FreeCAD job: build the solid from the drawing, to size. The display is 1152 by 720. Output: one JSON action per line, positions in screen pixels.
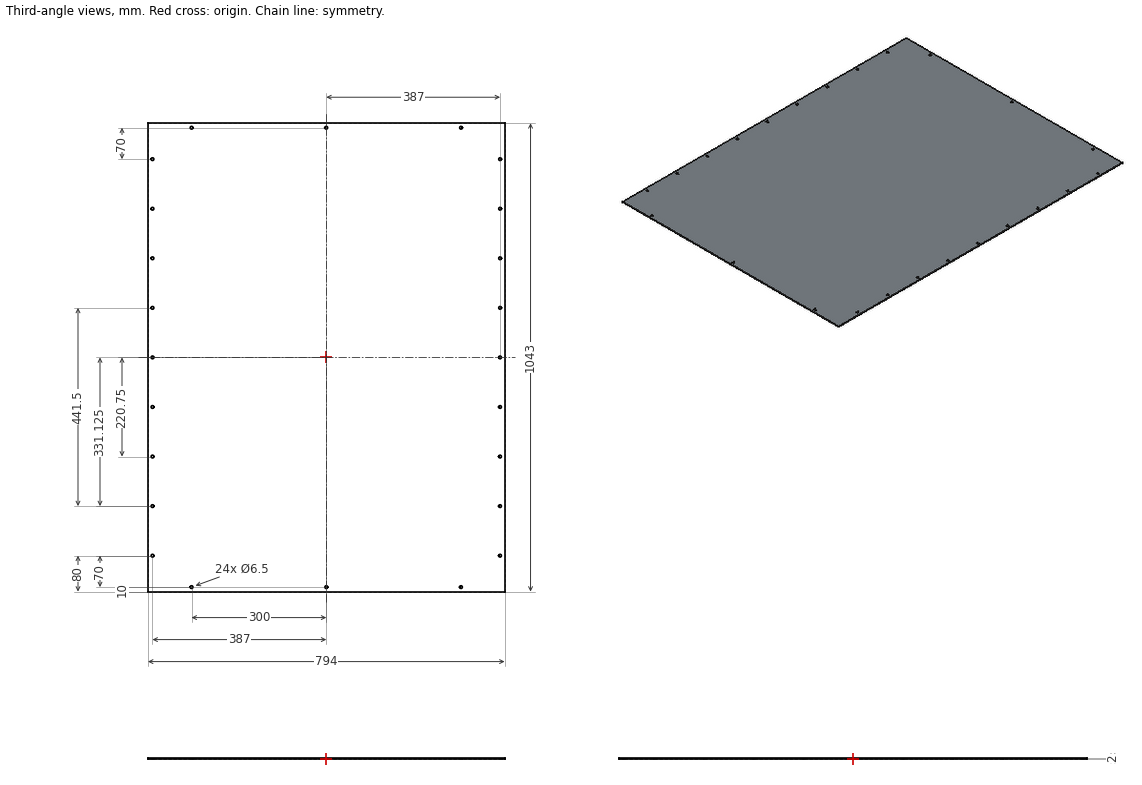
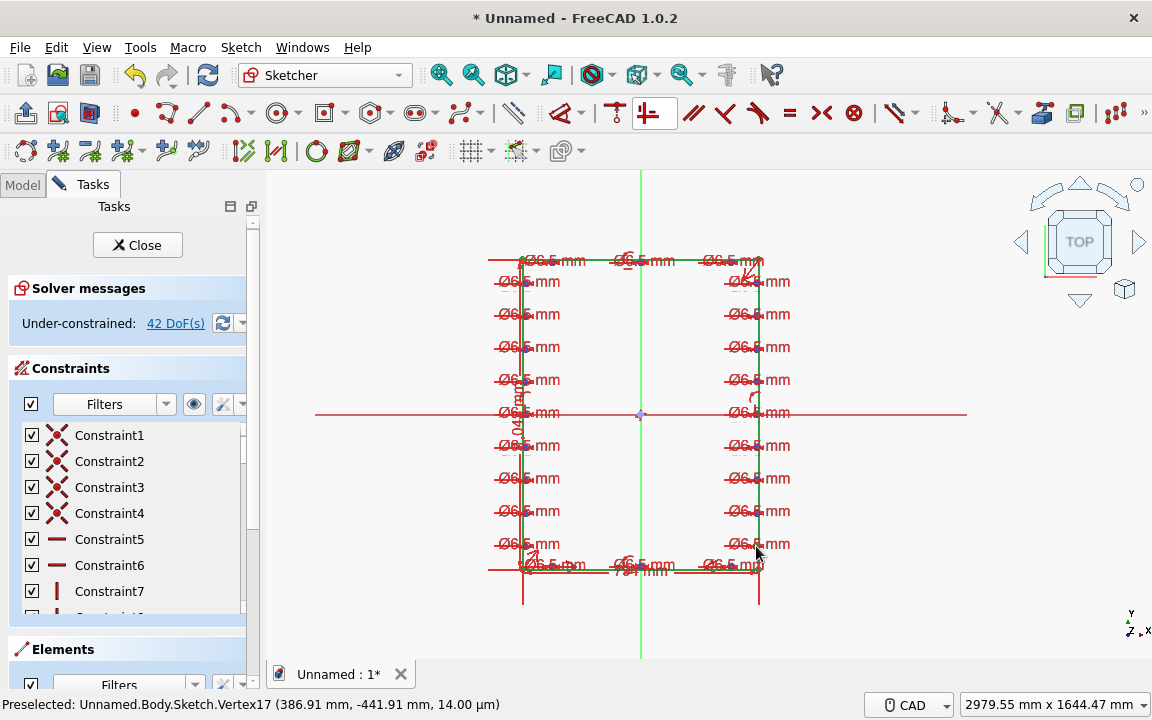
{"action": "left_click", "coordinate": [641, 600]}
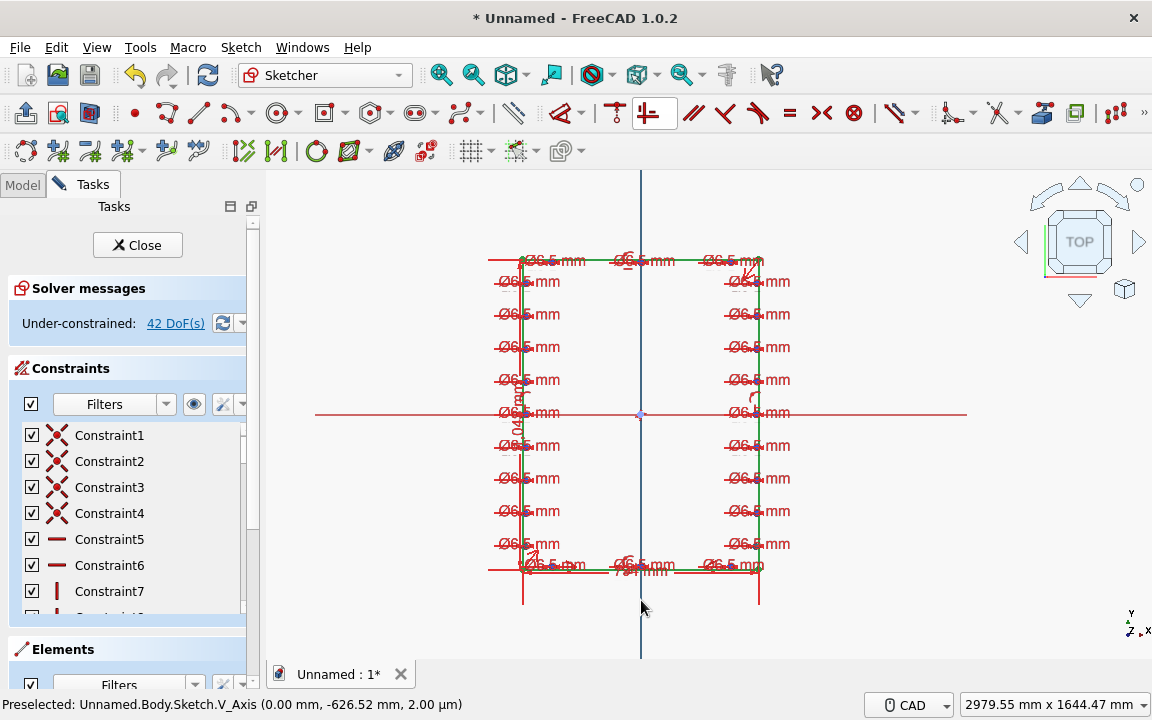
{"action": "left_click", "coordinate": [822, 114]}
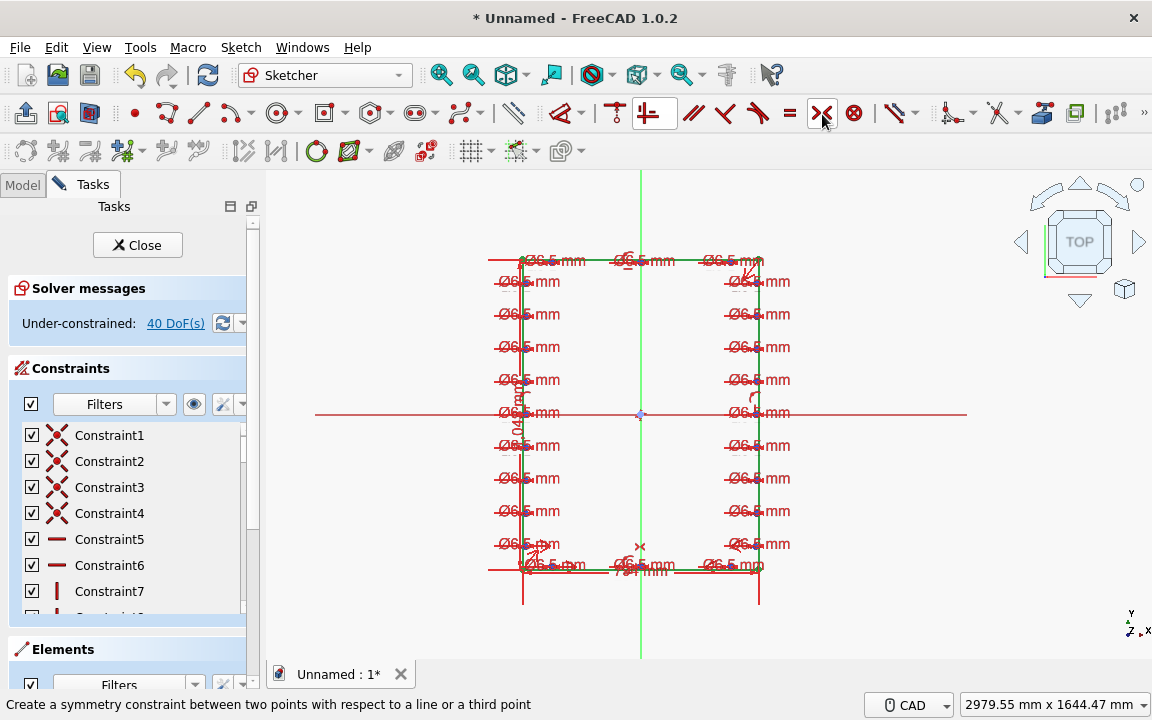
{"action": "left_click", "coordinate": [526, 513]}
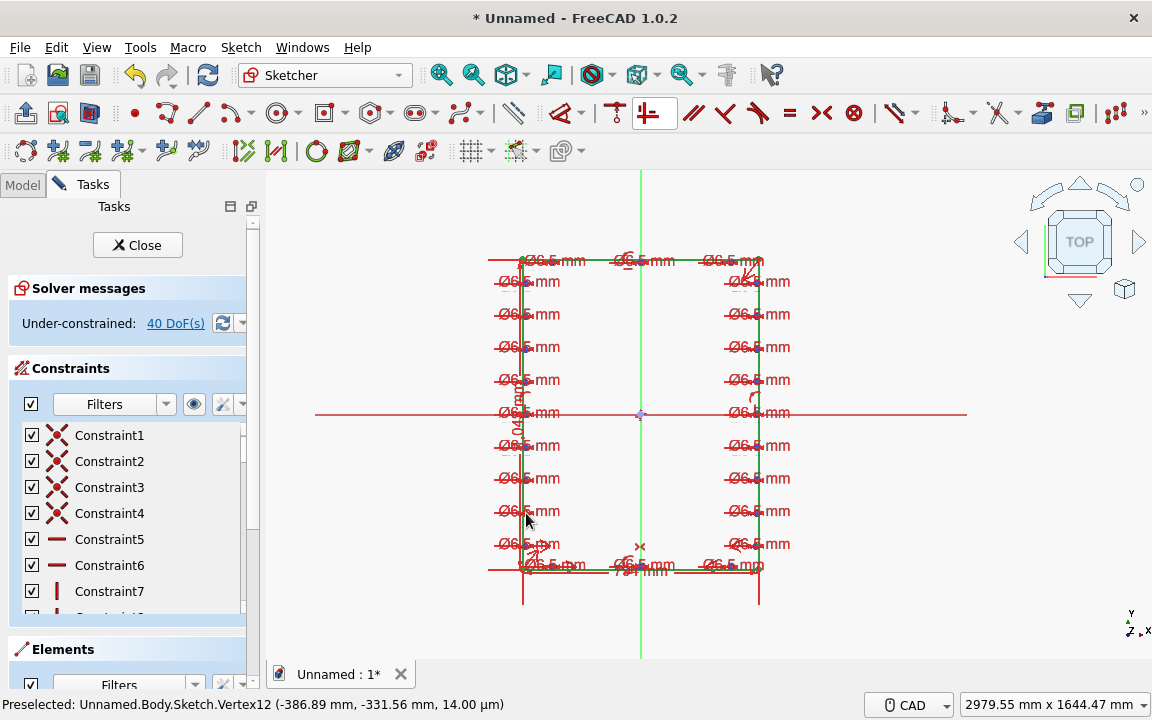
{"action": "left_click", "coordinate": [756, 513]}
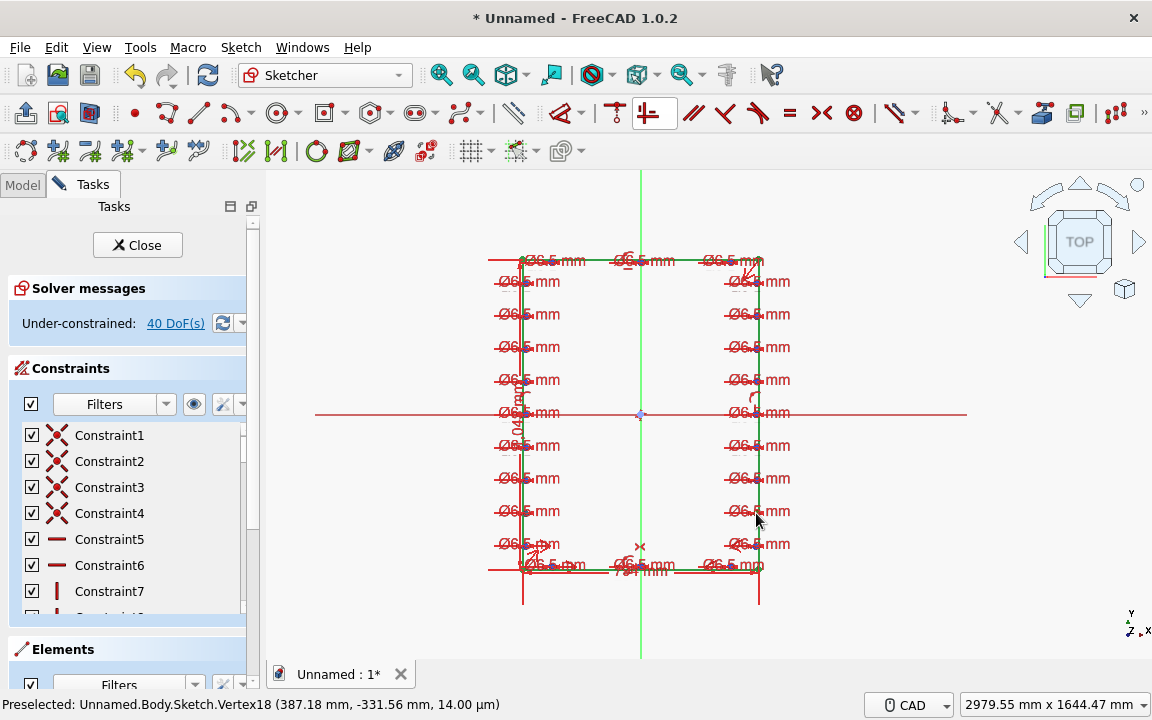
{"action": "left_click", "coordinate": [641, 600]}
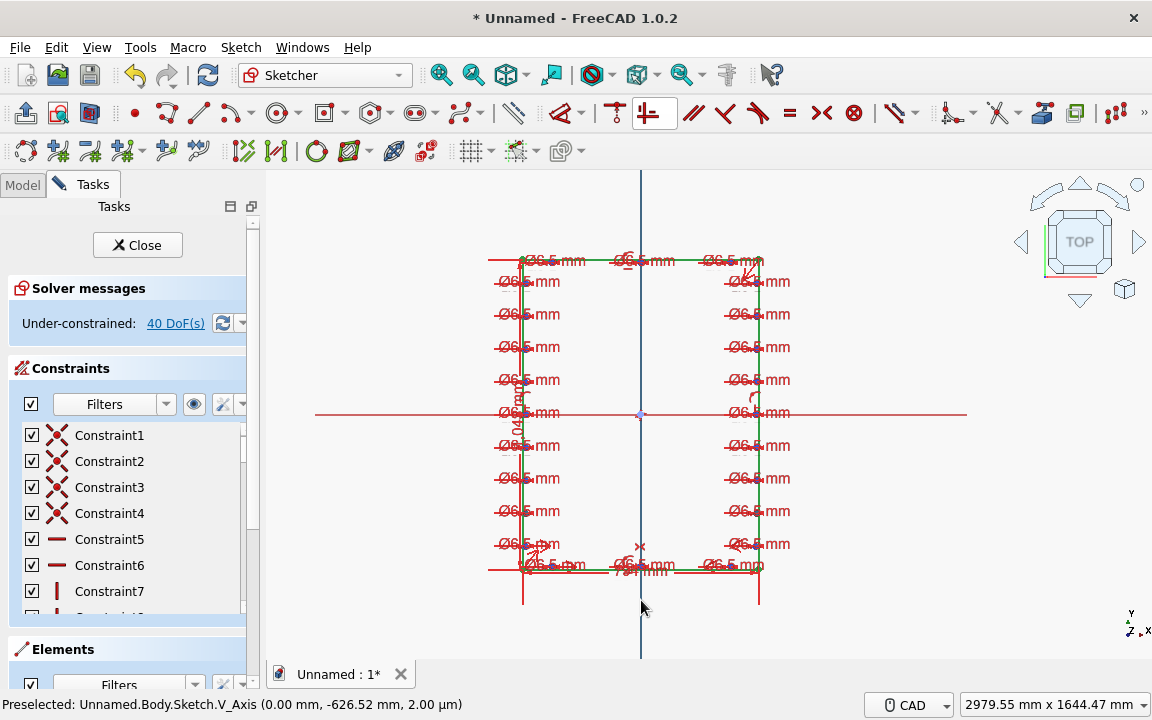
{"action": "left_click", "coordinate": [822, 114]}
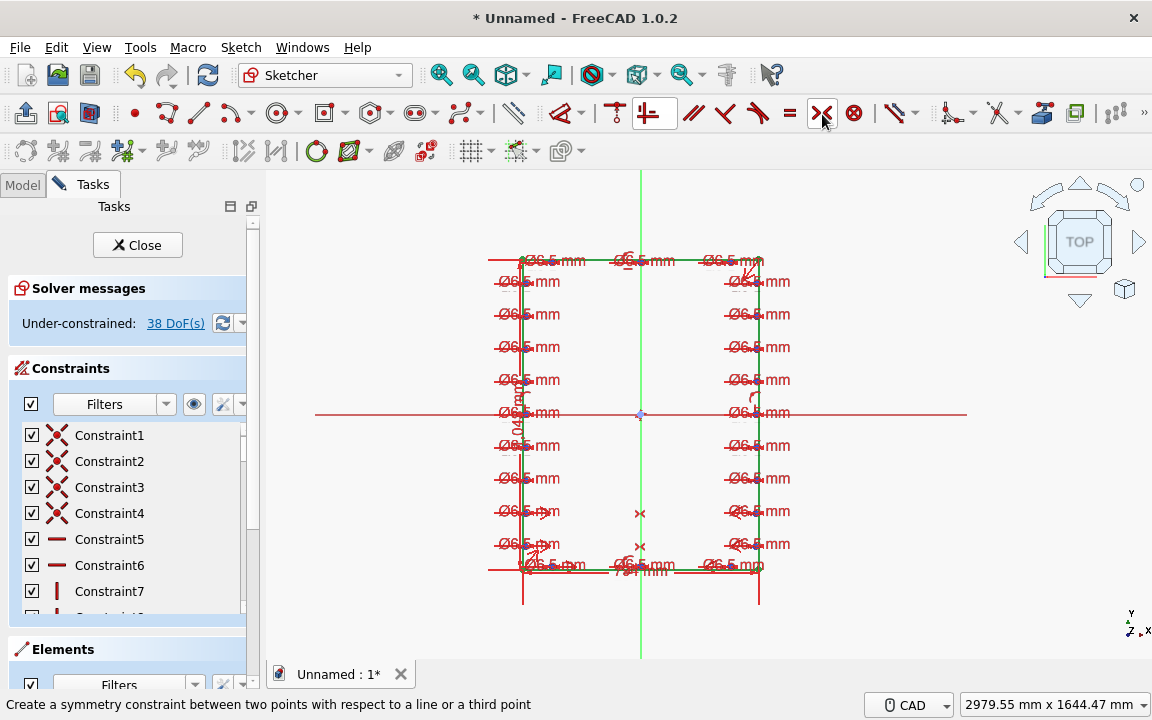
{"action": "left_click", "coordinate": [526, 480]}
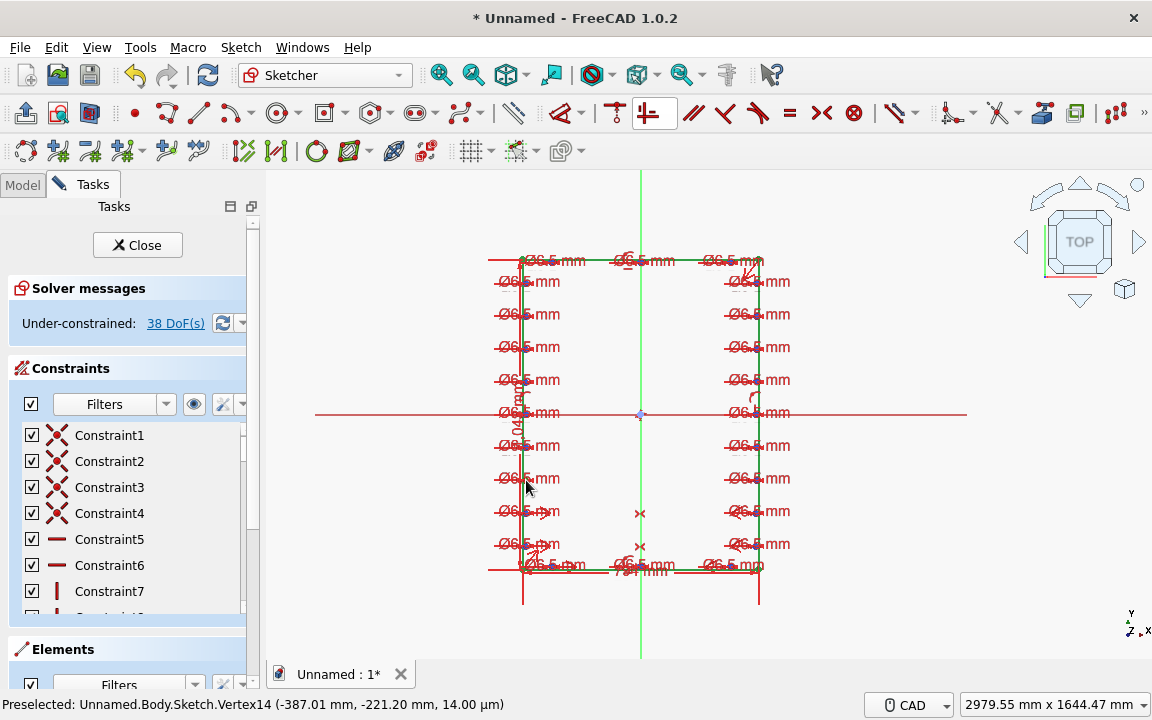
{"action": "left_click", "coordinate": [756, 480]}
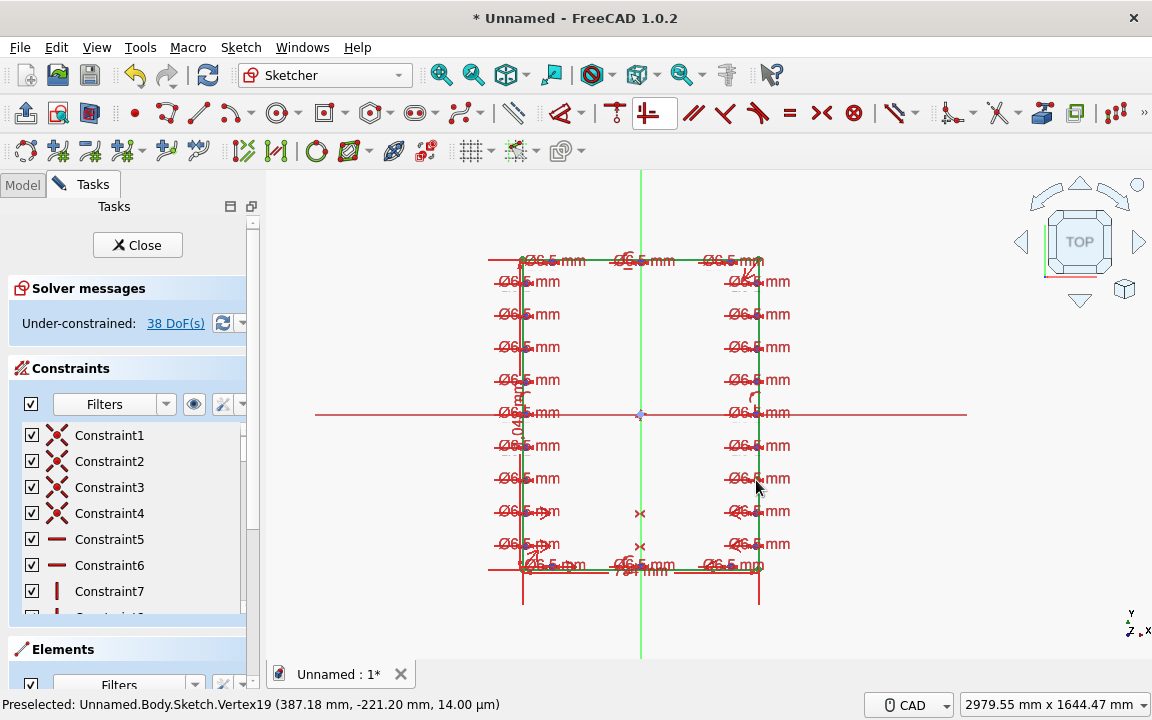
{"action": "left_click", "coordinate": [641, 600]}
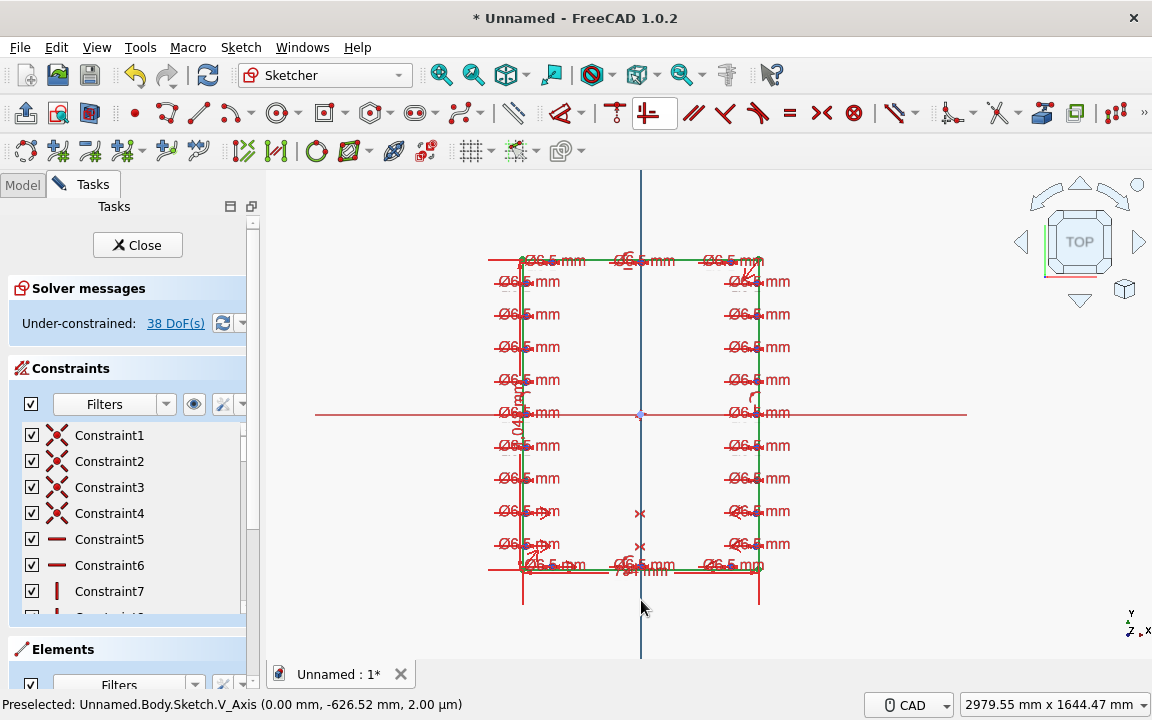
{"action": "left_click", "coordinate": [822, 114]}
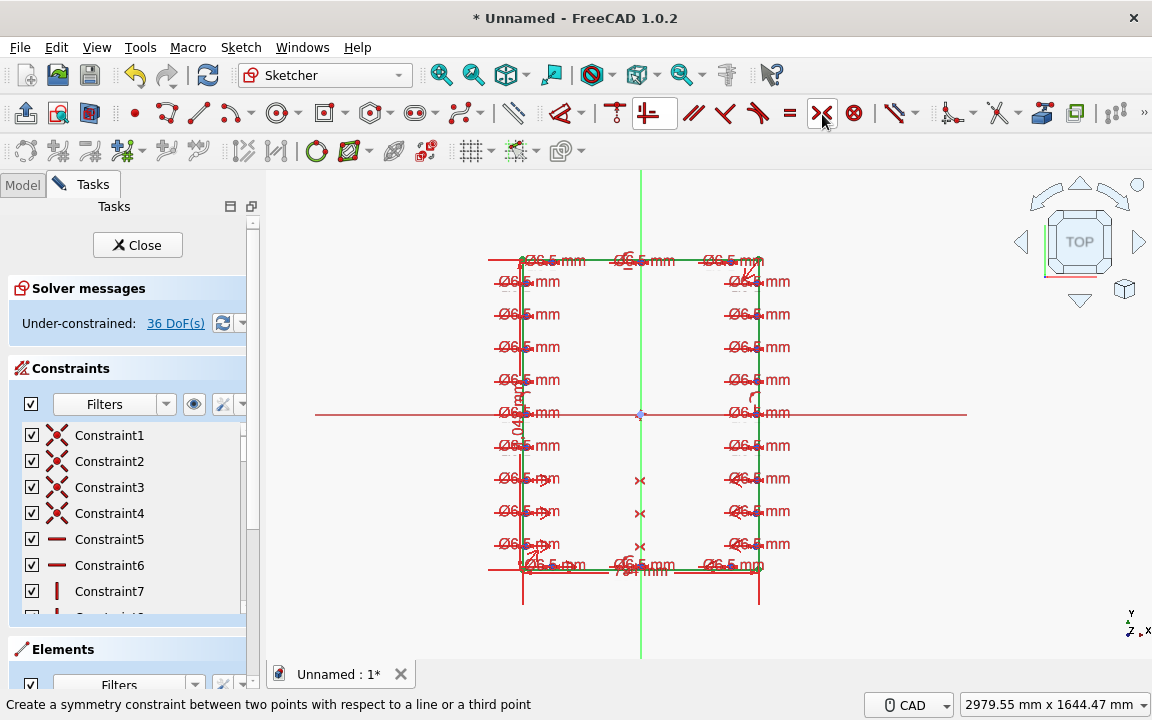
{"action": "left_click", "coordinate": [526, 448]}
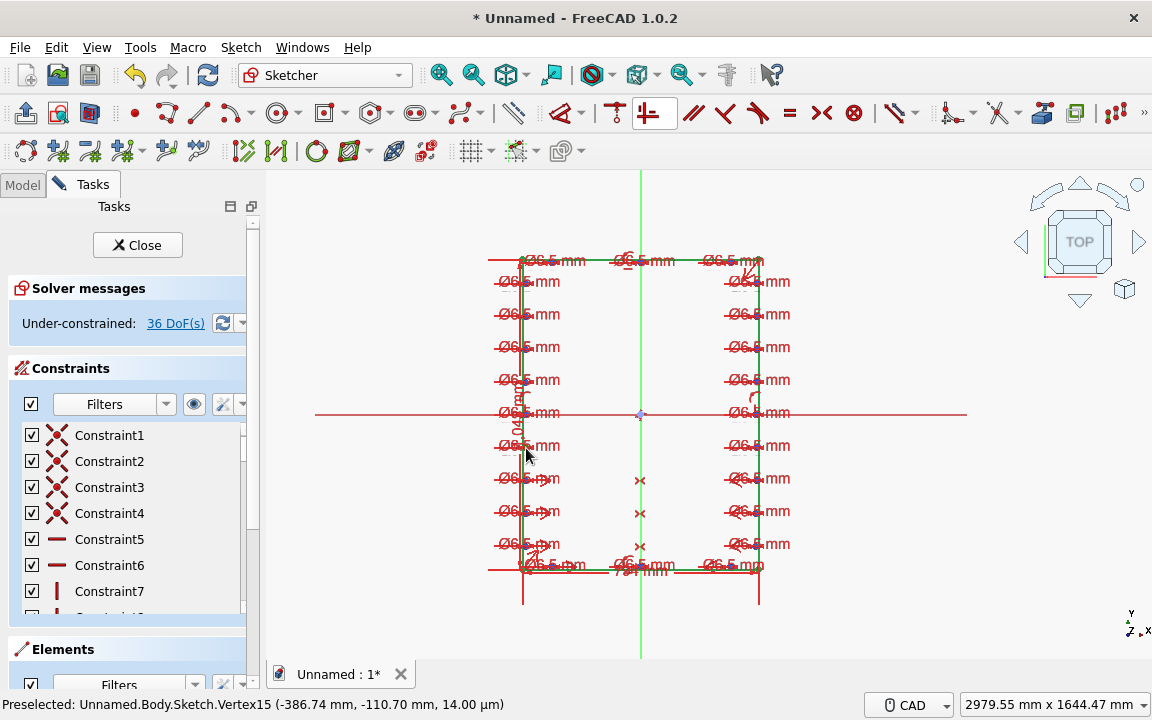
{"action": "left_click", "coordinate": [756, 448]}